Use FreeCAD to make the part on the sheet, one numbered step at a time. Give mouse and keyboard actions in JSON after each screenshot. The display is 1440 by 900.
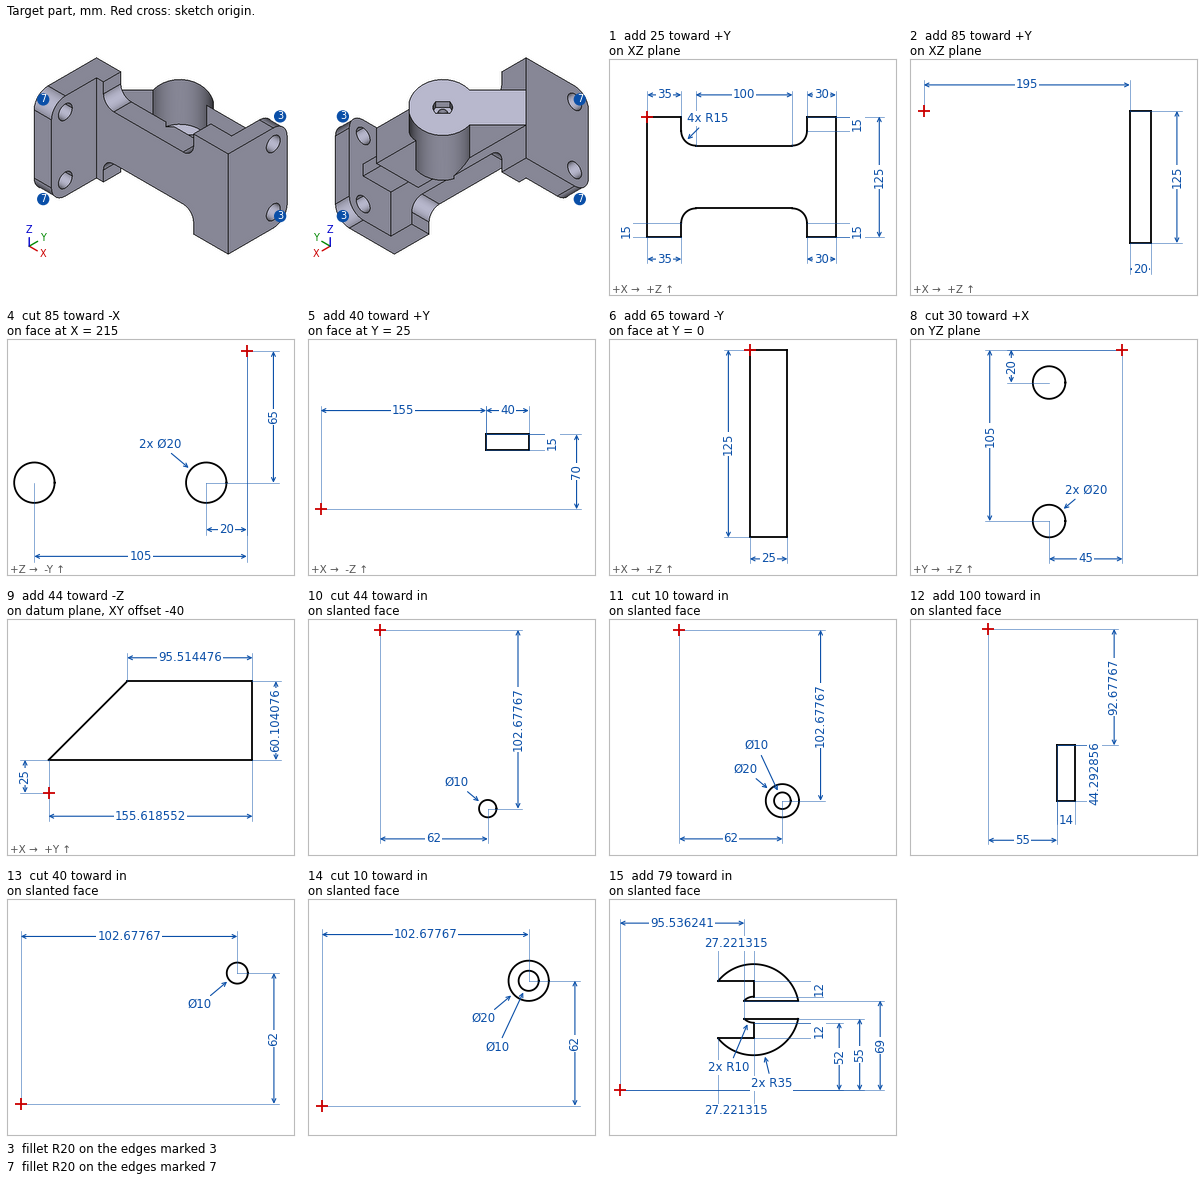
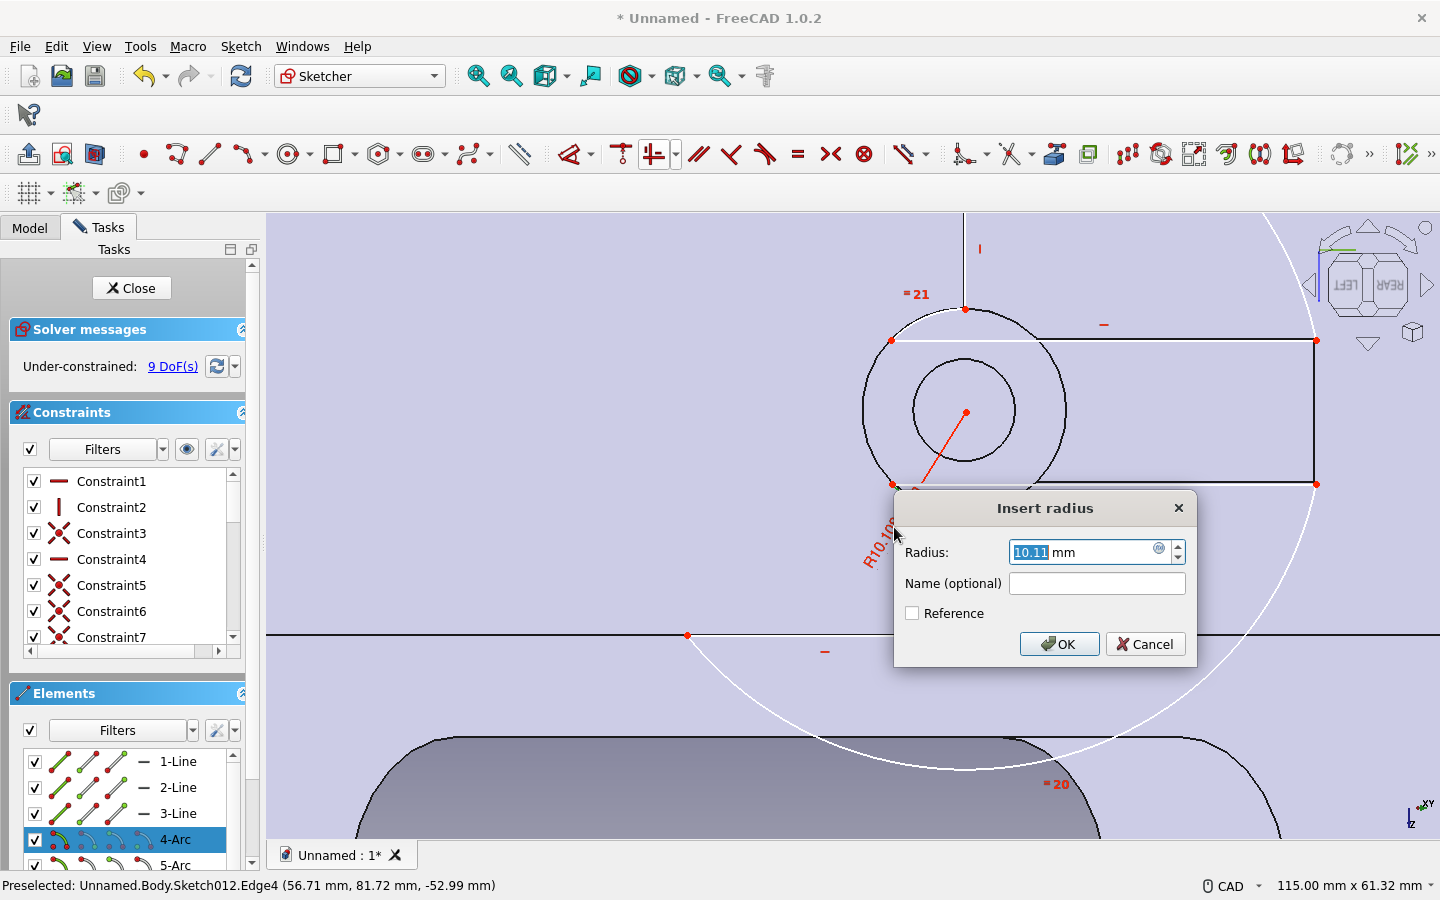
{"action": "type", "text": "10"}
{"action": "key", "text": "Return"}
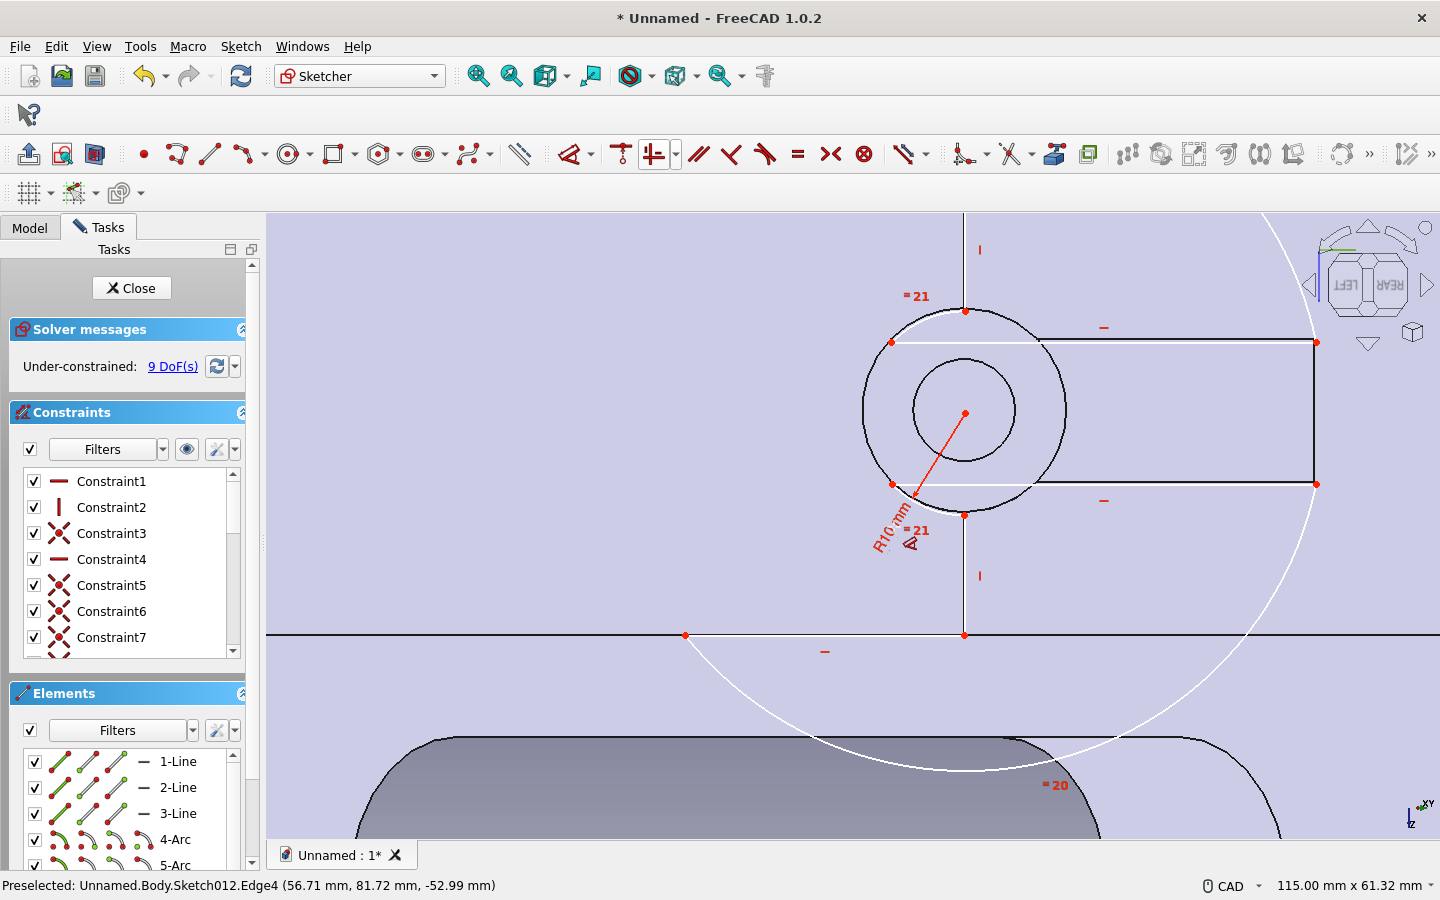
{"action": "left_click", "coordinate": [888, 763]}
{"action": "left_click", "coordinate": [881, 794]}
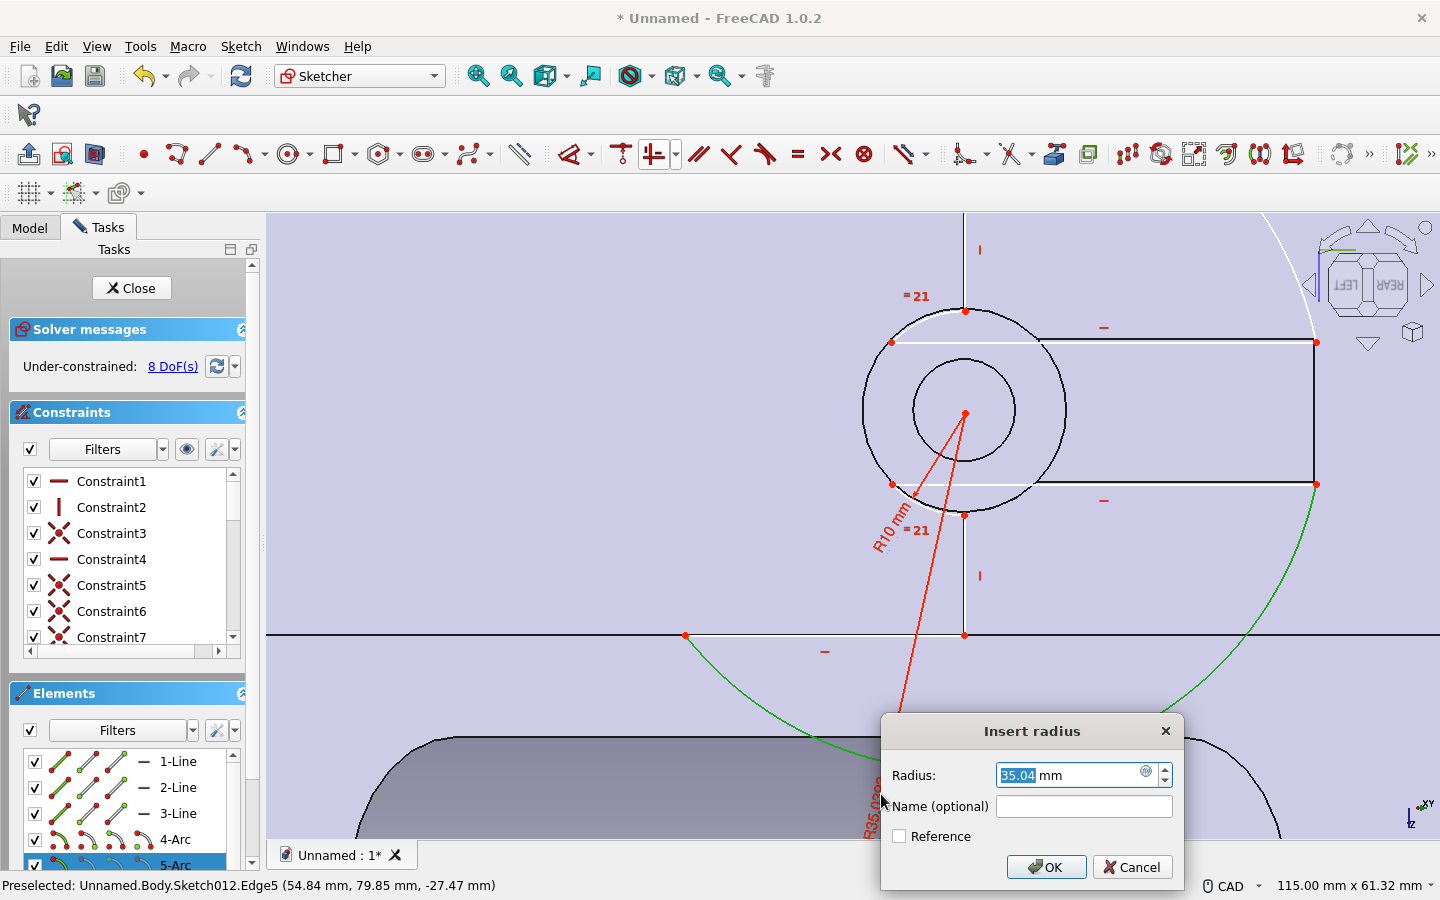
{"action": "type", "text": "35"}
{"action": "key", "text": "Return"}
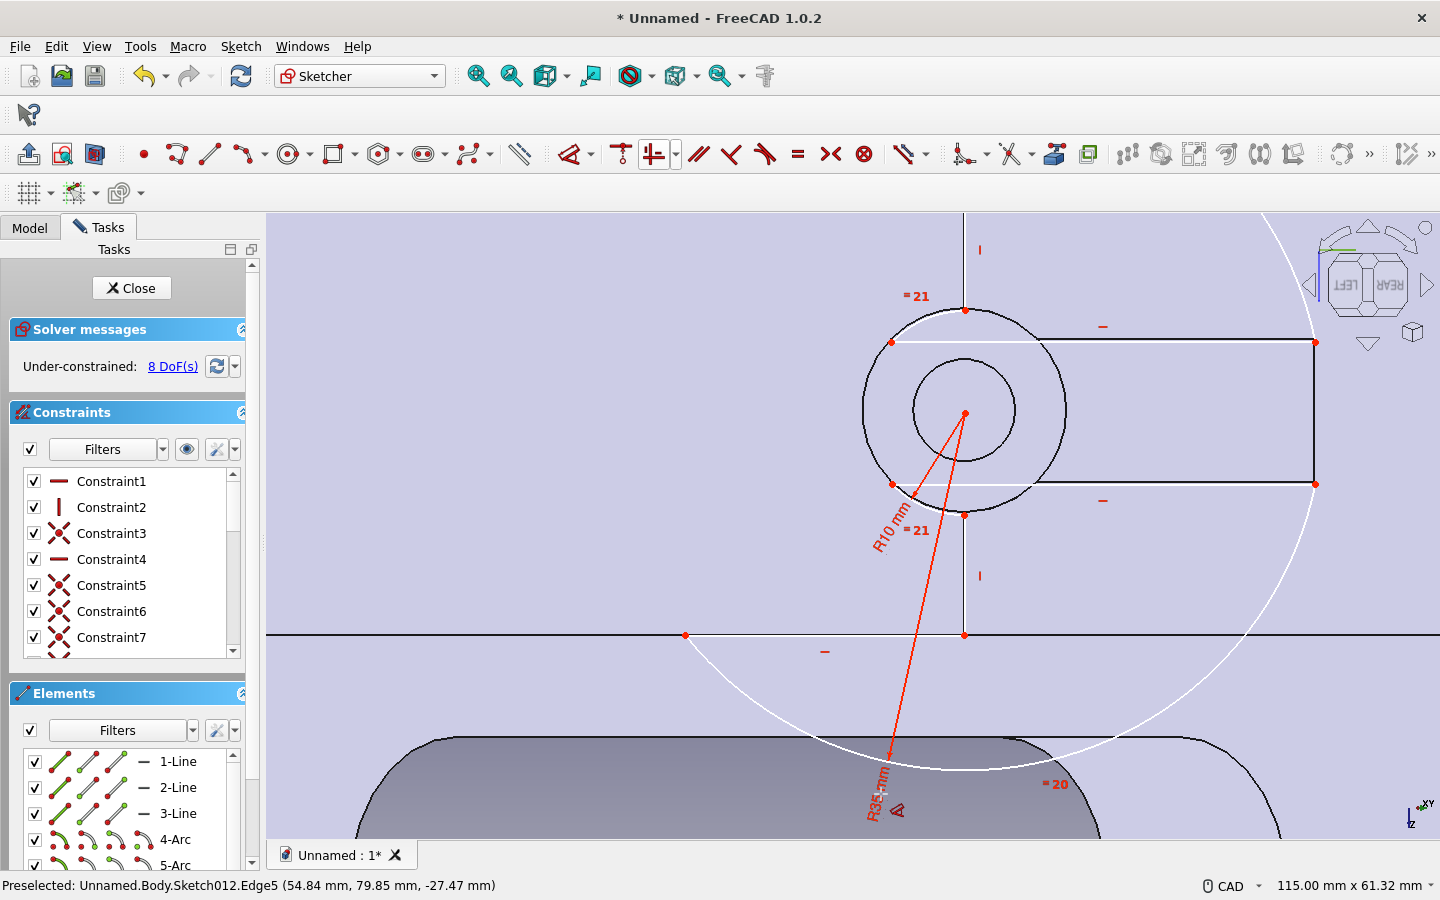
{"action": "left_click", "coordinate": [965, 551]}
{"action": "left_click", "coordinate": [999, 575]}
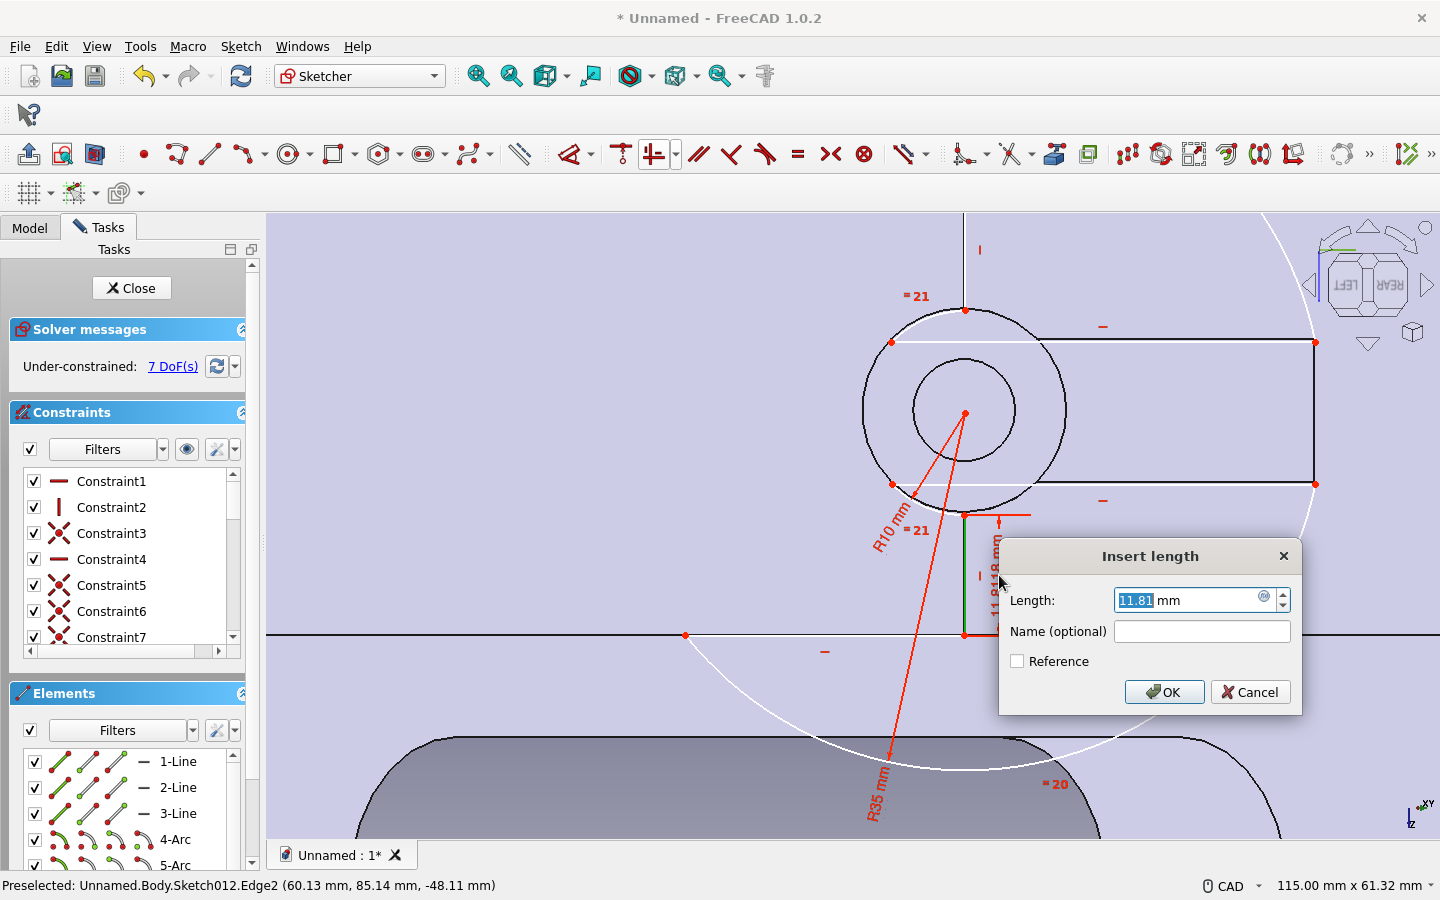
{"action": "type", "text": "12"}
{"action": "key", "text": "Return"}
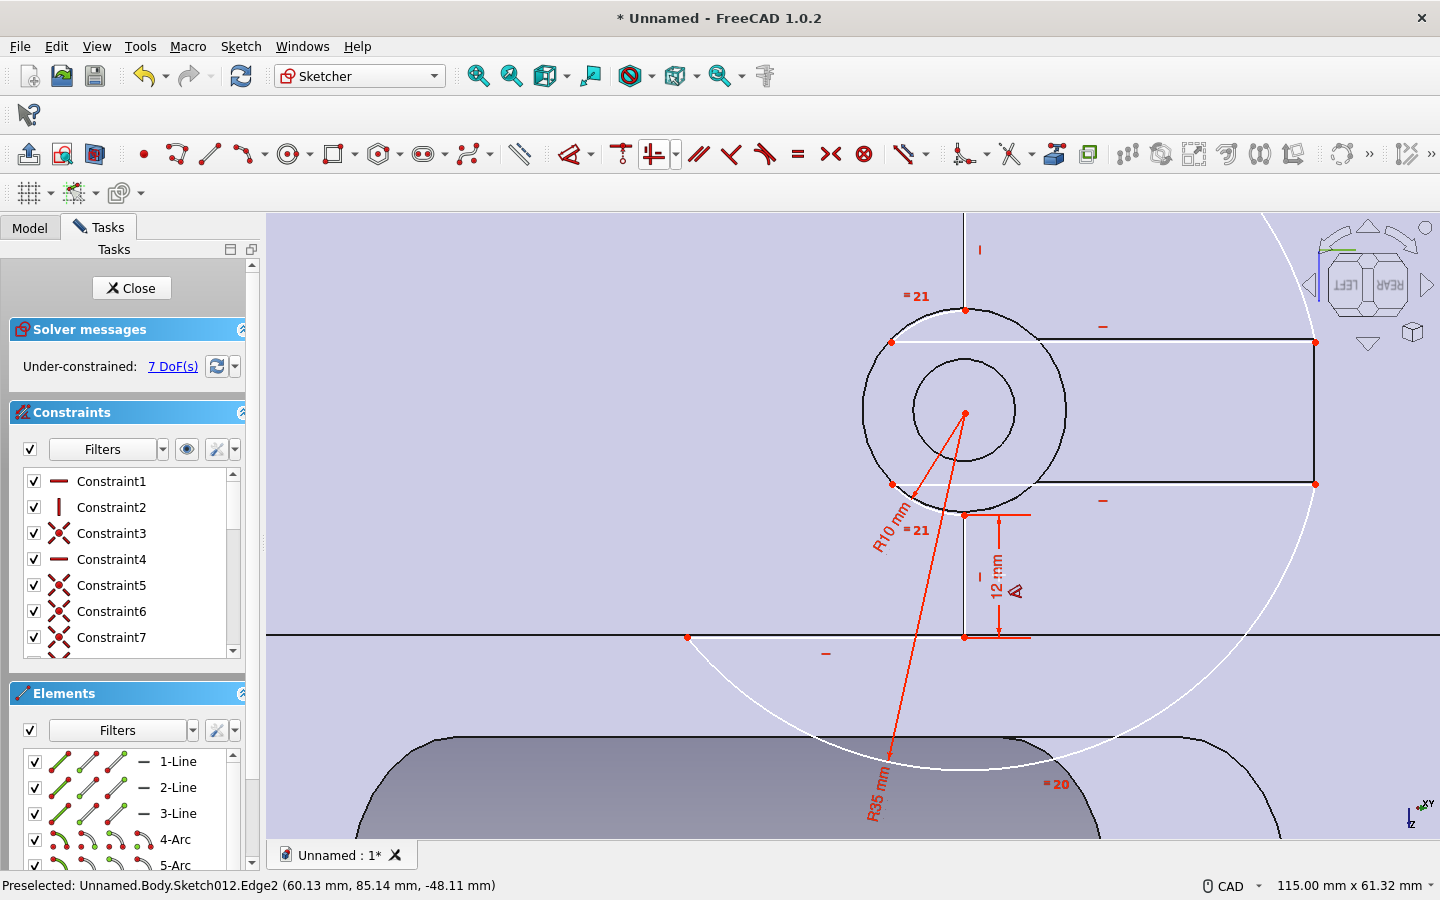
{"action": "left_click", "coordinate": [965, 274]}
{"action": "left_click", "coordinate": [999, 276]}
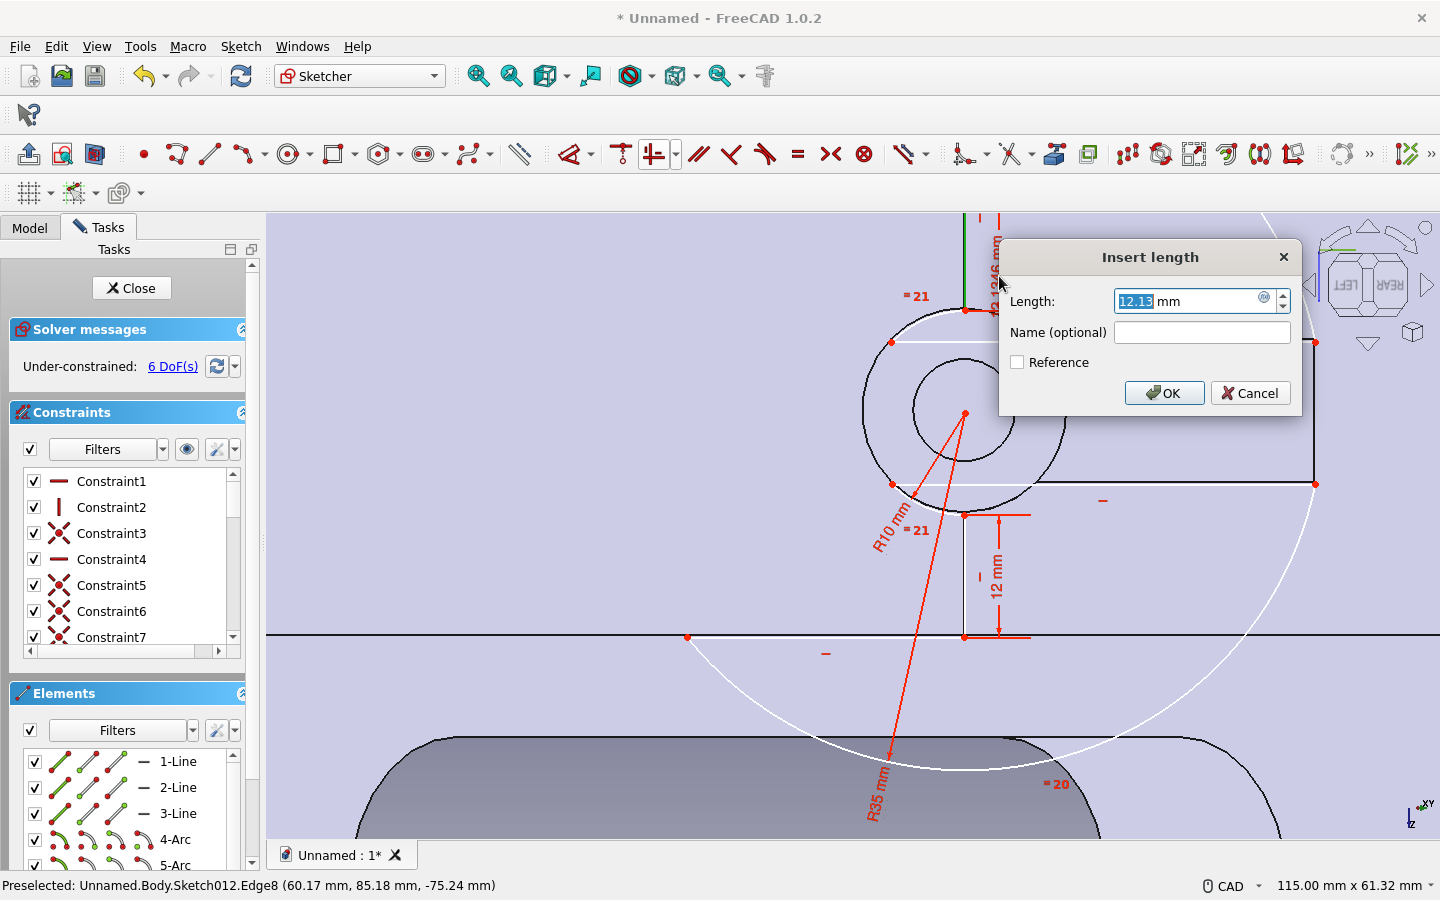
{"action": "type", "text": "12"}
{"action": "key", "text": "Return"}